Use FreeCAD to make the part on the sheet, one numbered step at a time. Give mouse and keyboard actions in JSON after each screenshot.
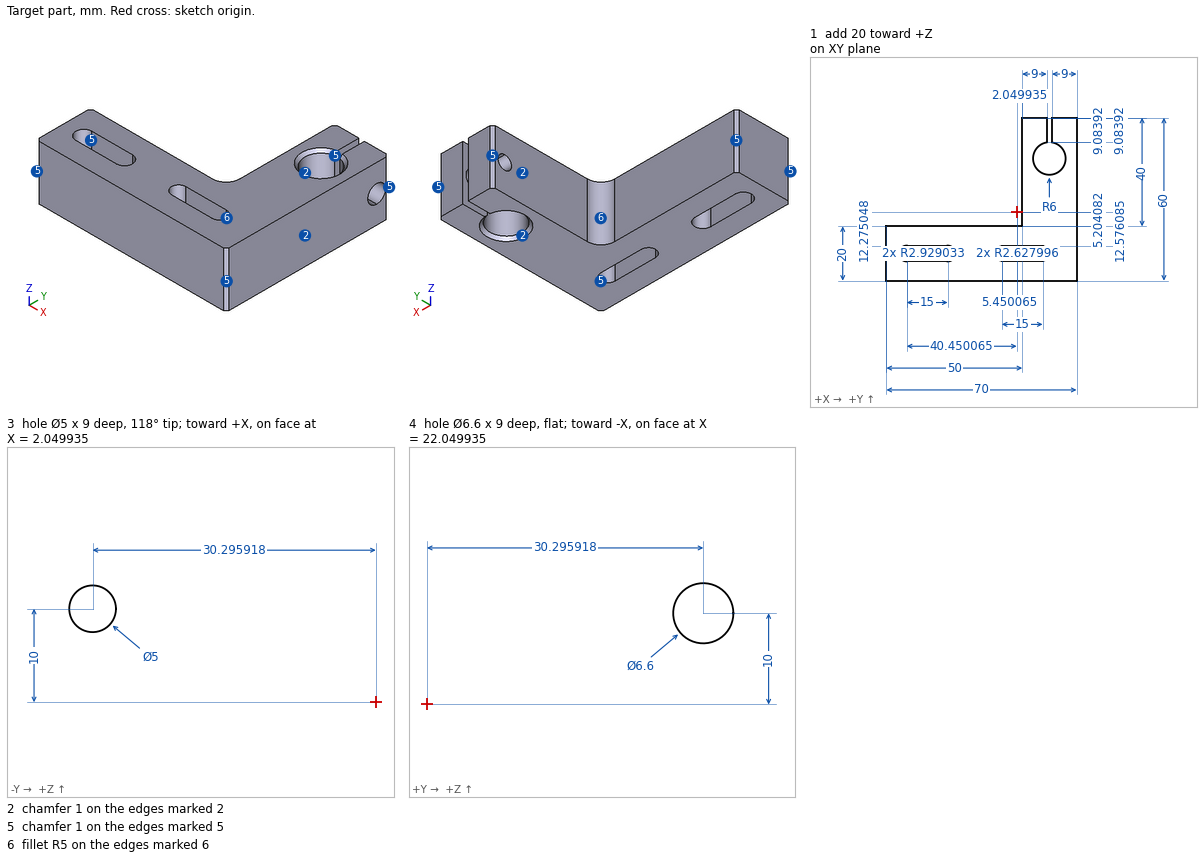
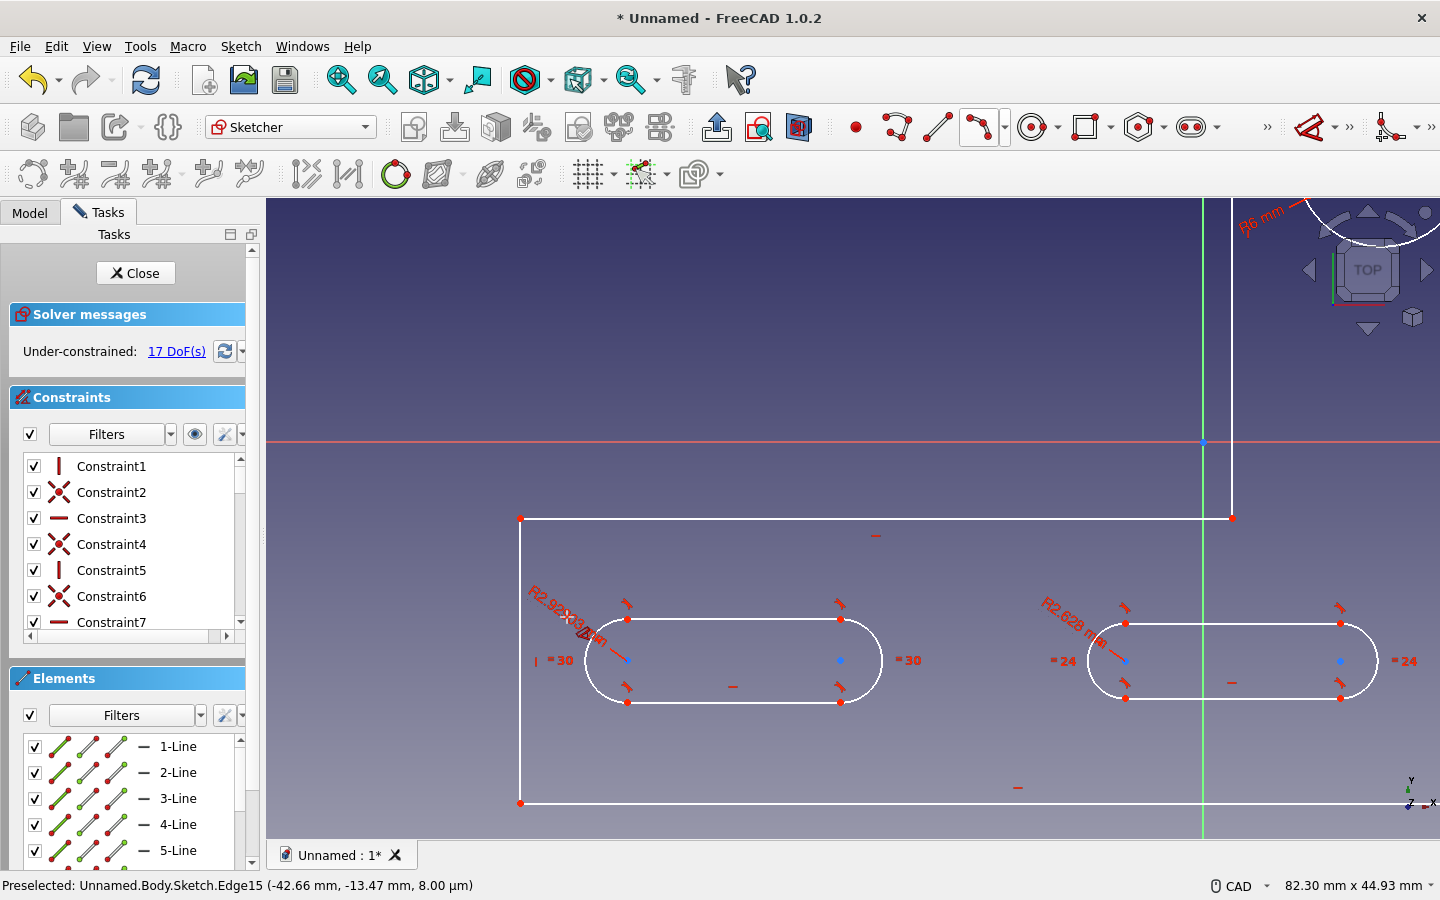
{"action": "scroll", "coordinate": [593, 637], "scroll_direction": "down", "scroll_amount": 4}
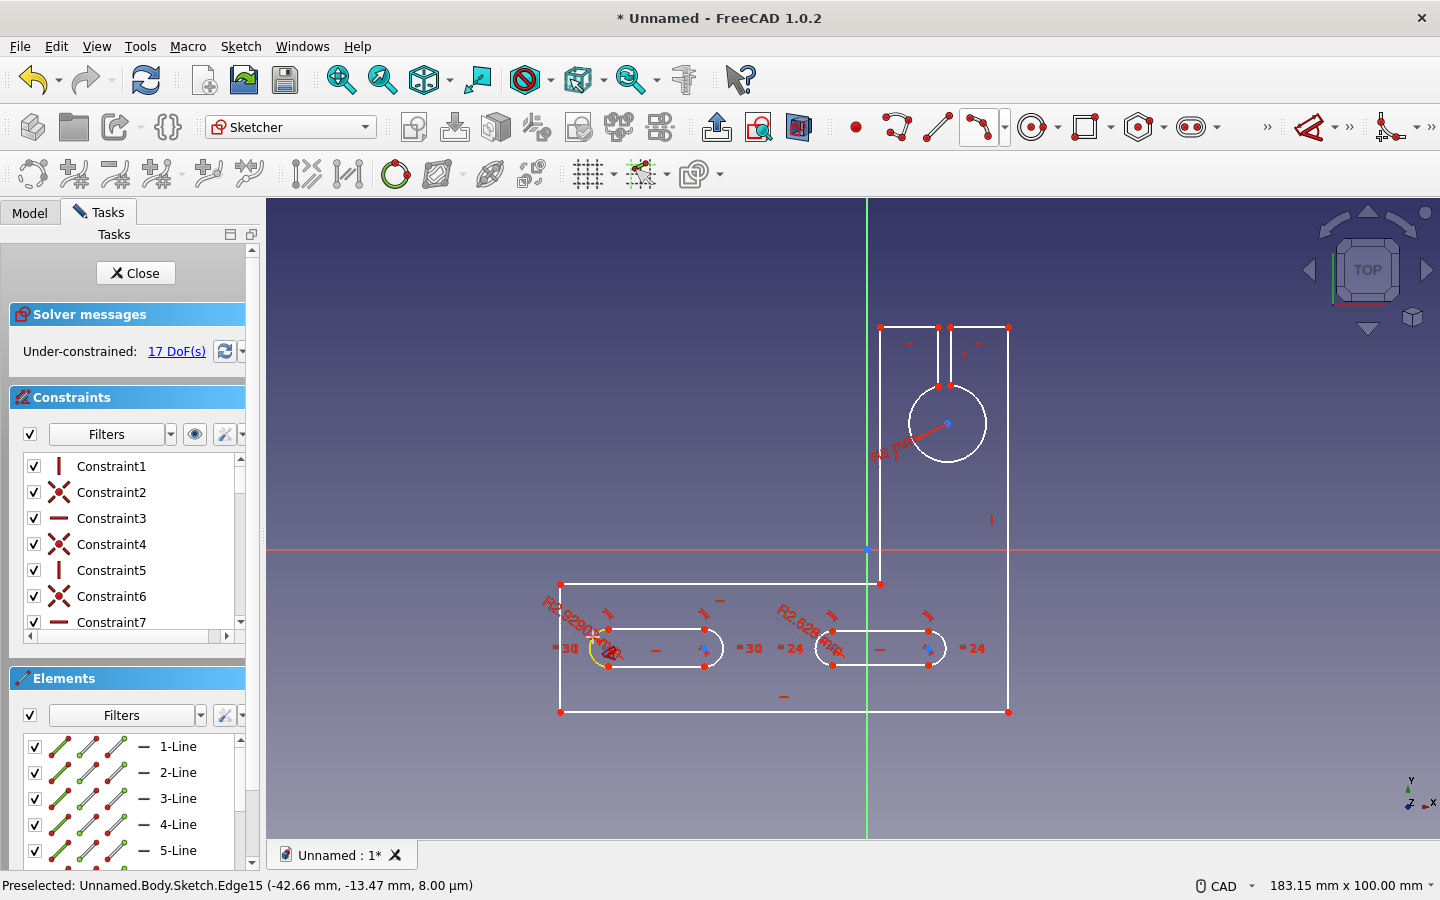
{"action": "left_click", "coordinate": [921, 327]}
{"action": "left_click", "coordinate": [909, 293]}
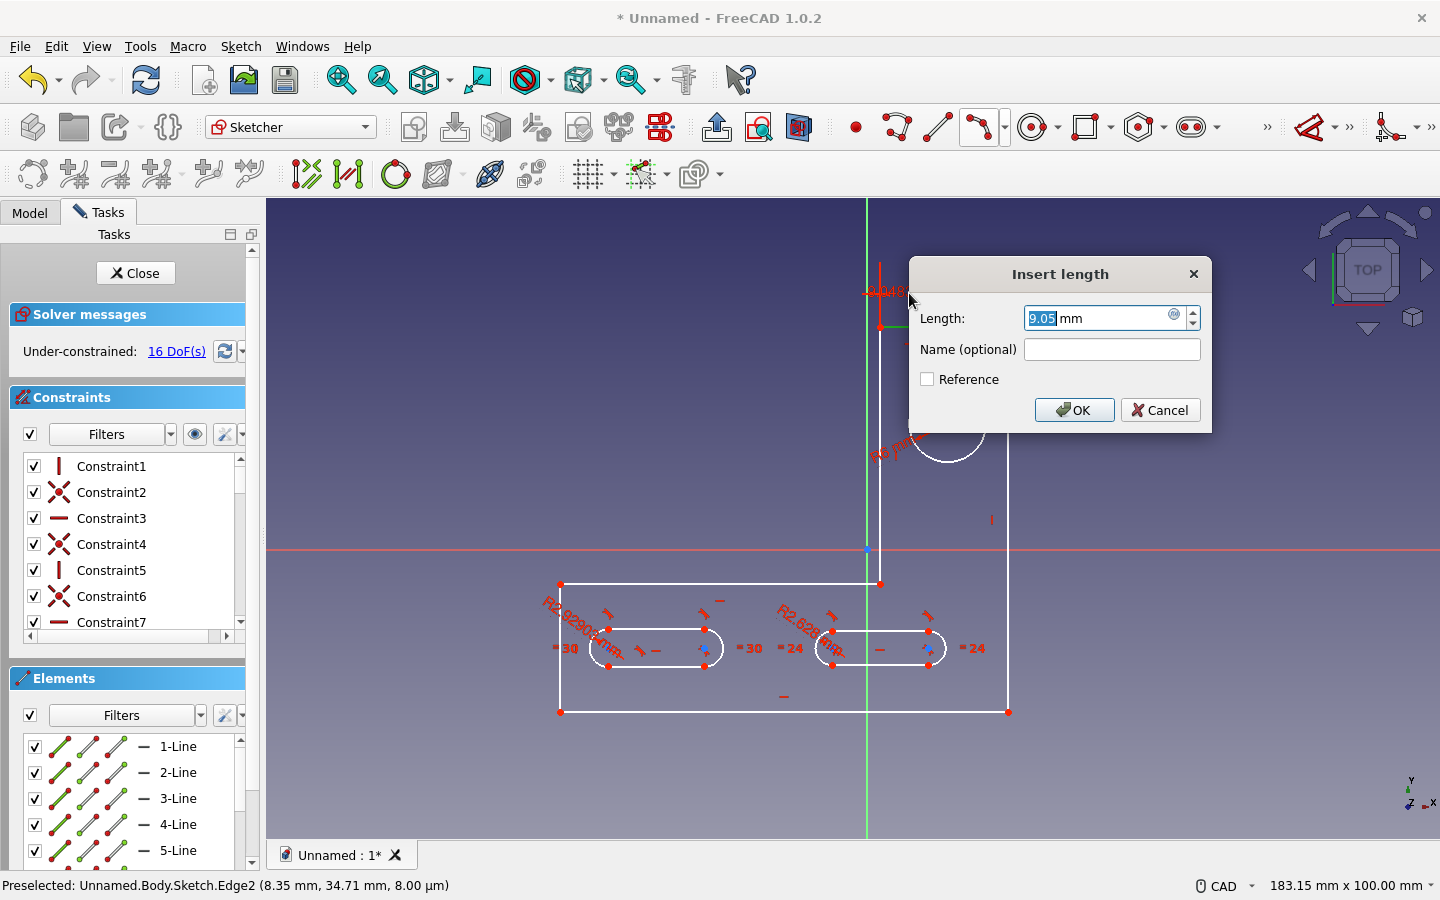
{"action": "type", "text": "9"}
{"action": "key", "text": "Return"}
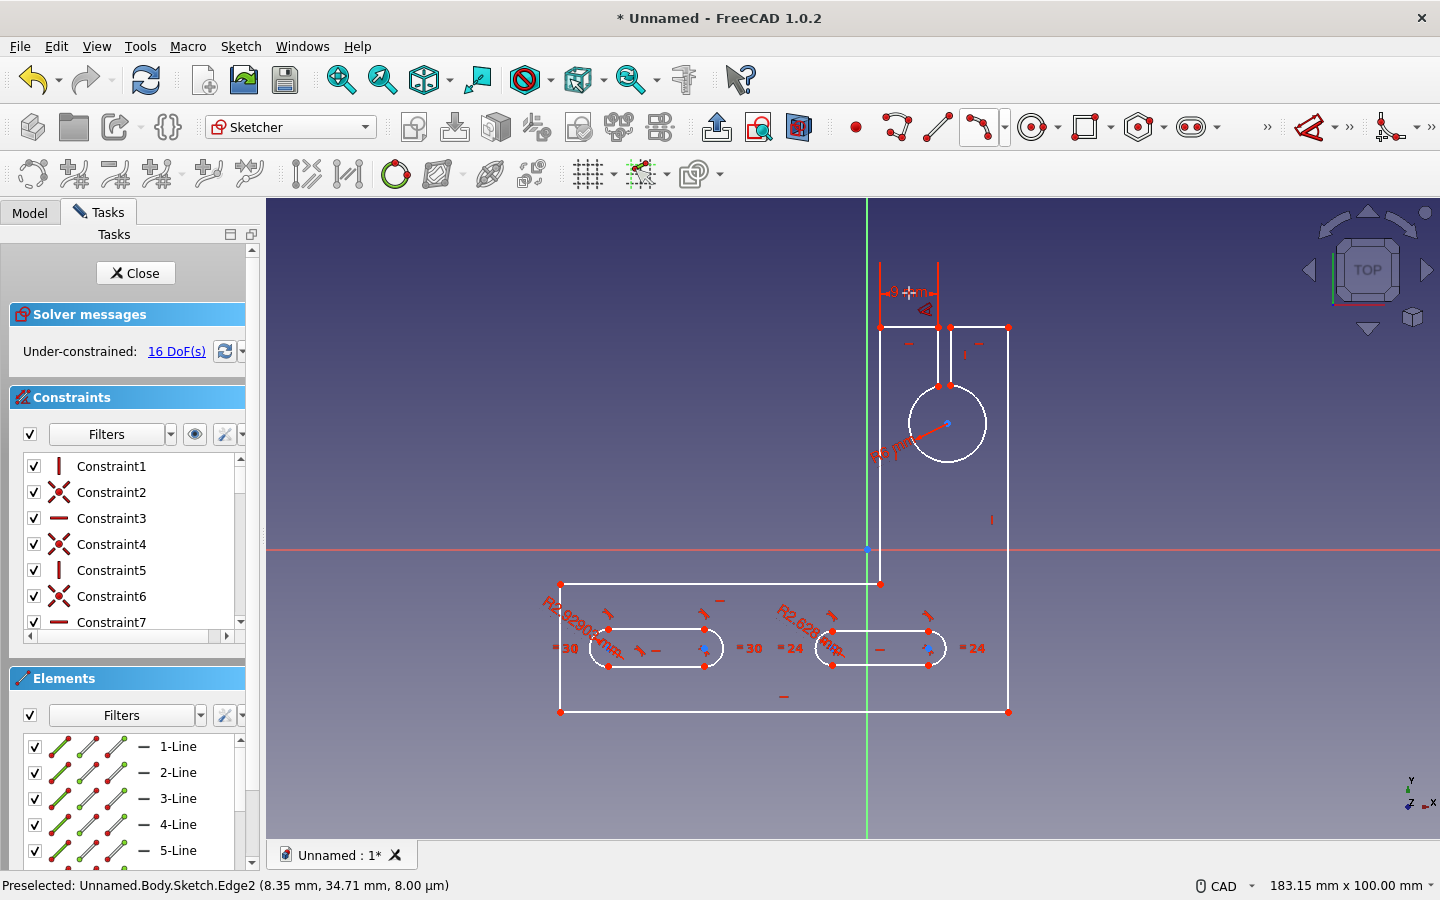
{"action": "left_click", "coordinate": [991, 327]}
{"action": "left_click", "coordinate": [980, 293]}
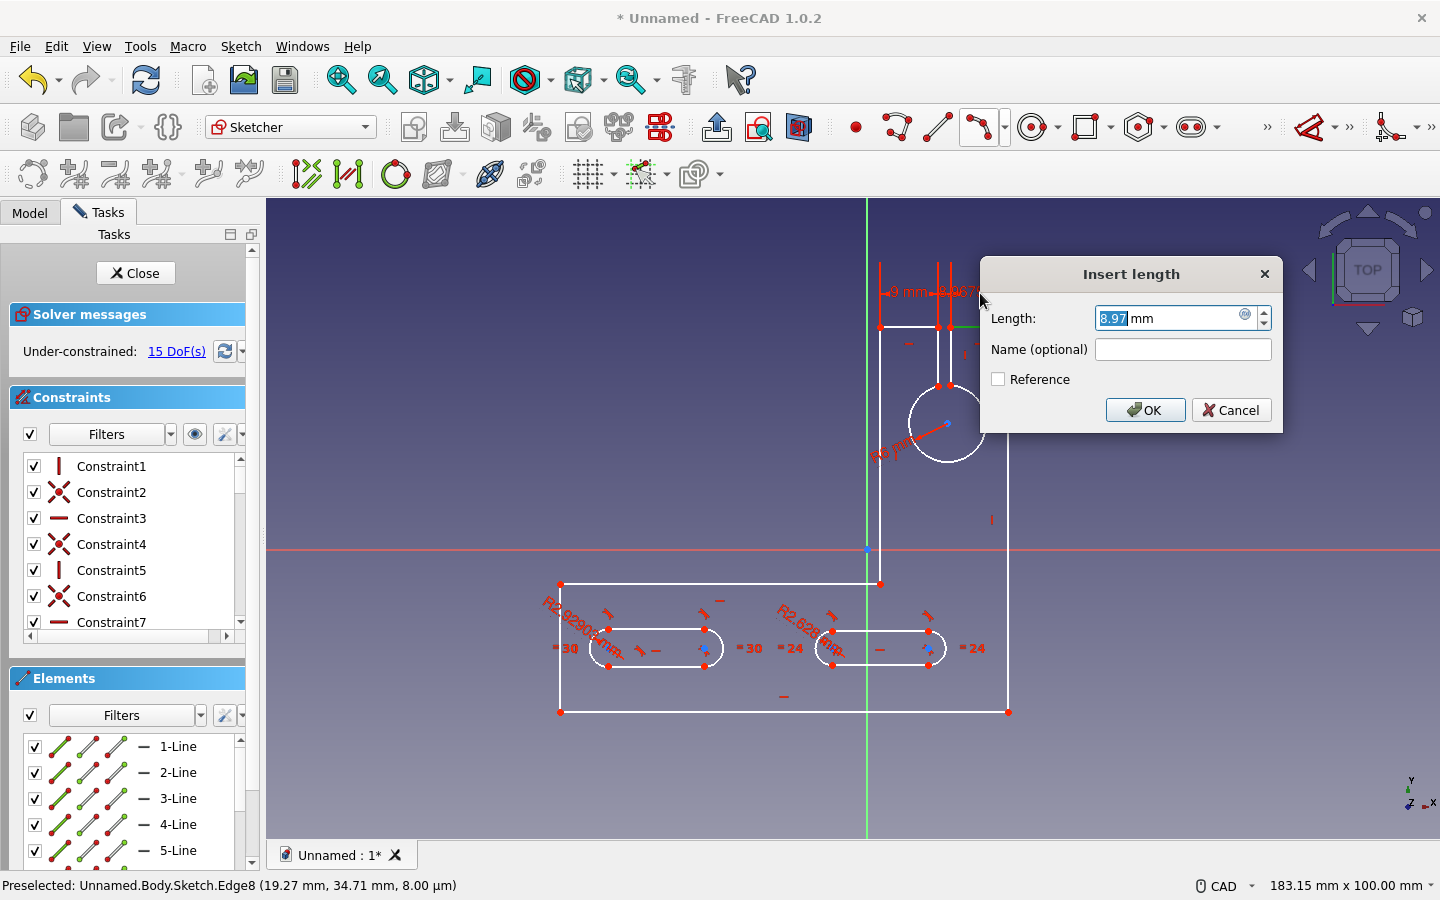
{"action": "type", "text": "9"}
{"action": "key", "text": "Return"}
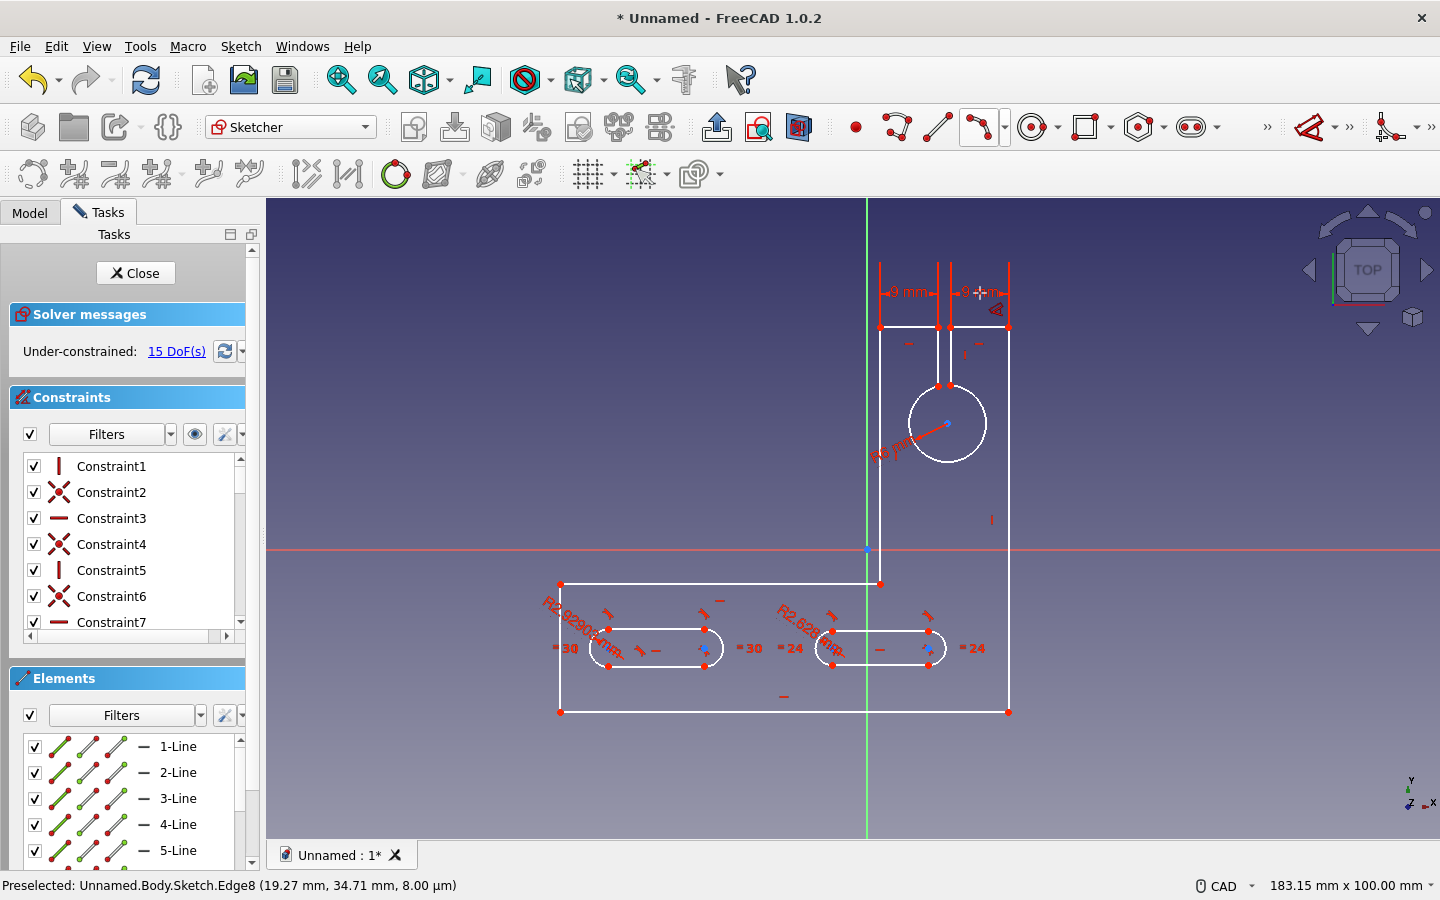
{"action": "left_click", "coordinate": [880, 404]}
{"action": "left_click", "coordinate": [914, 515]}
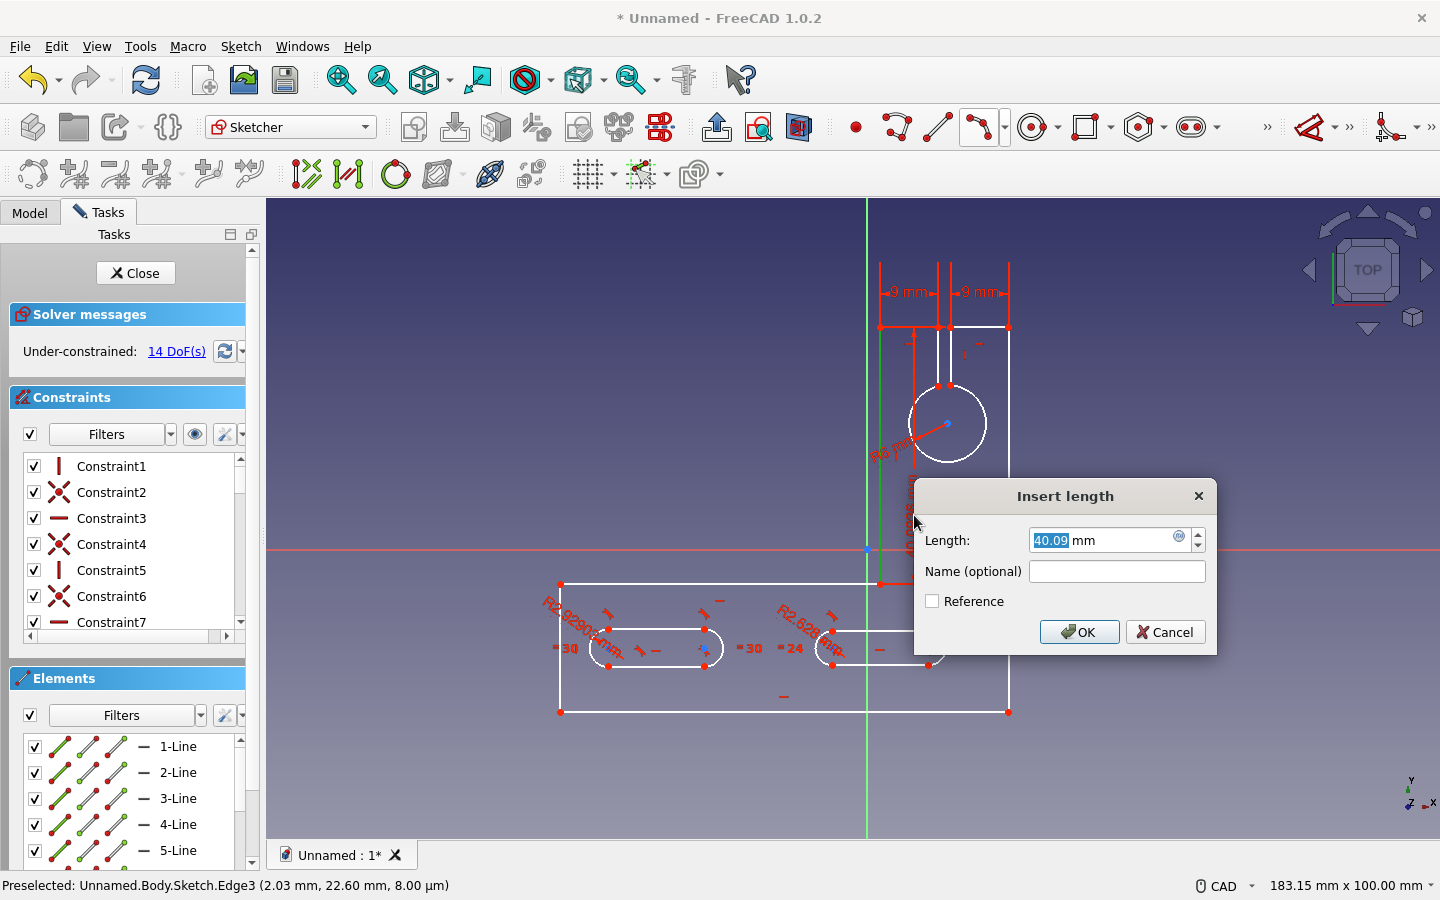
{"action": "type", "text": "40"}
{"action": "key", "text": "Return"}